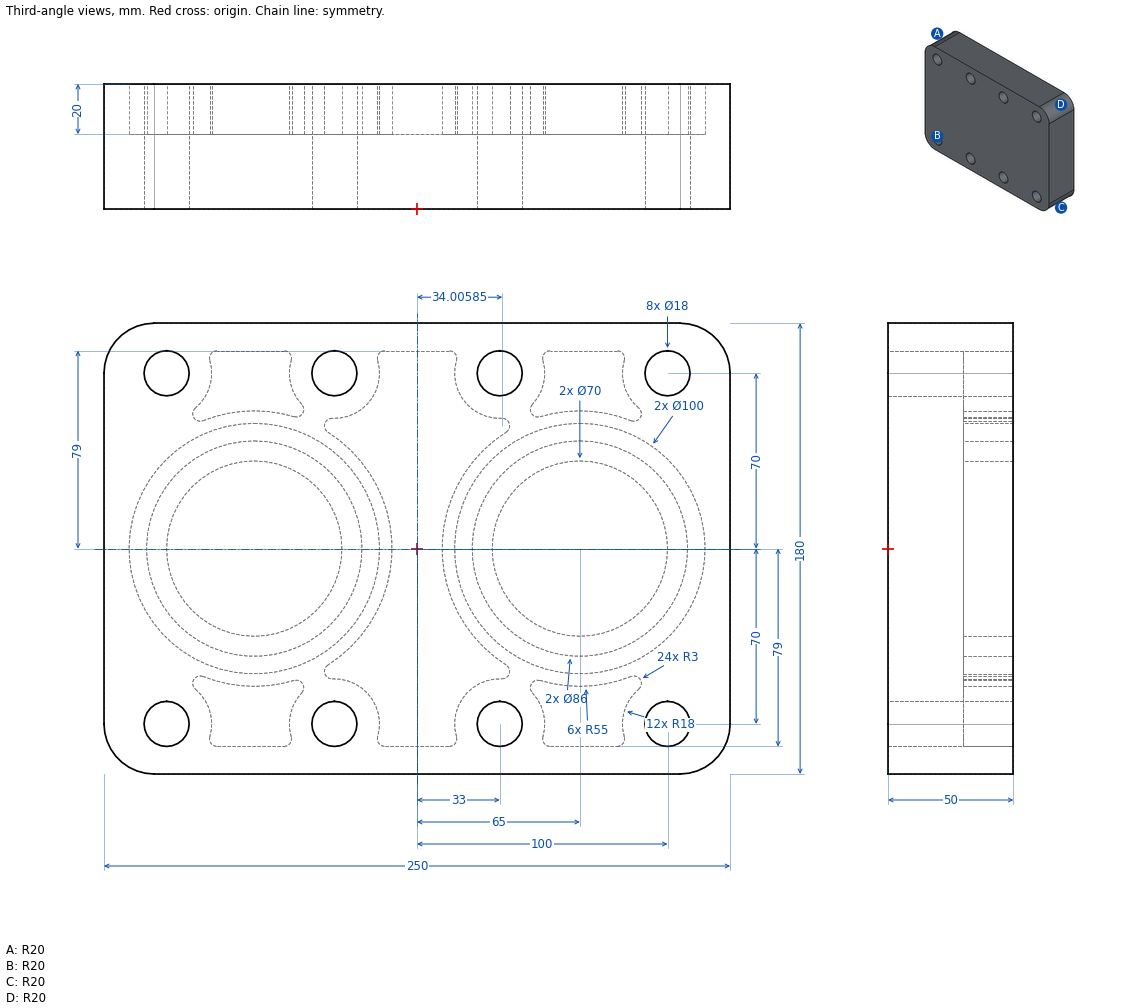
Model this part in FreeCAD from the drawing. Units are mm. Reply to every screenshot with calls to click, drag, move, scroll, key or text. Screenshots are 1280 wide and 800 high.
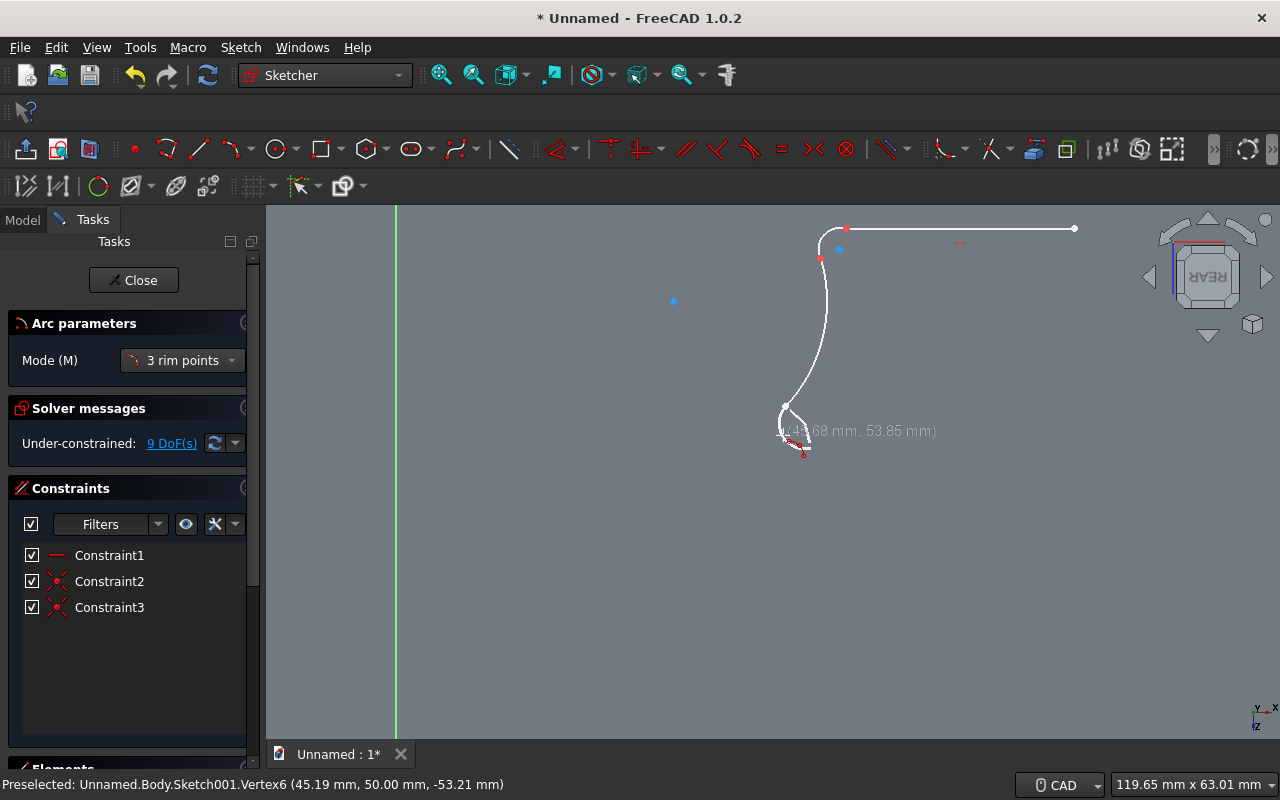
click(783, 435)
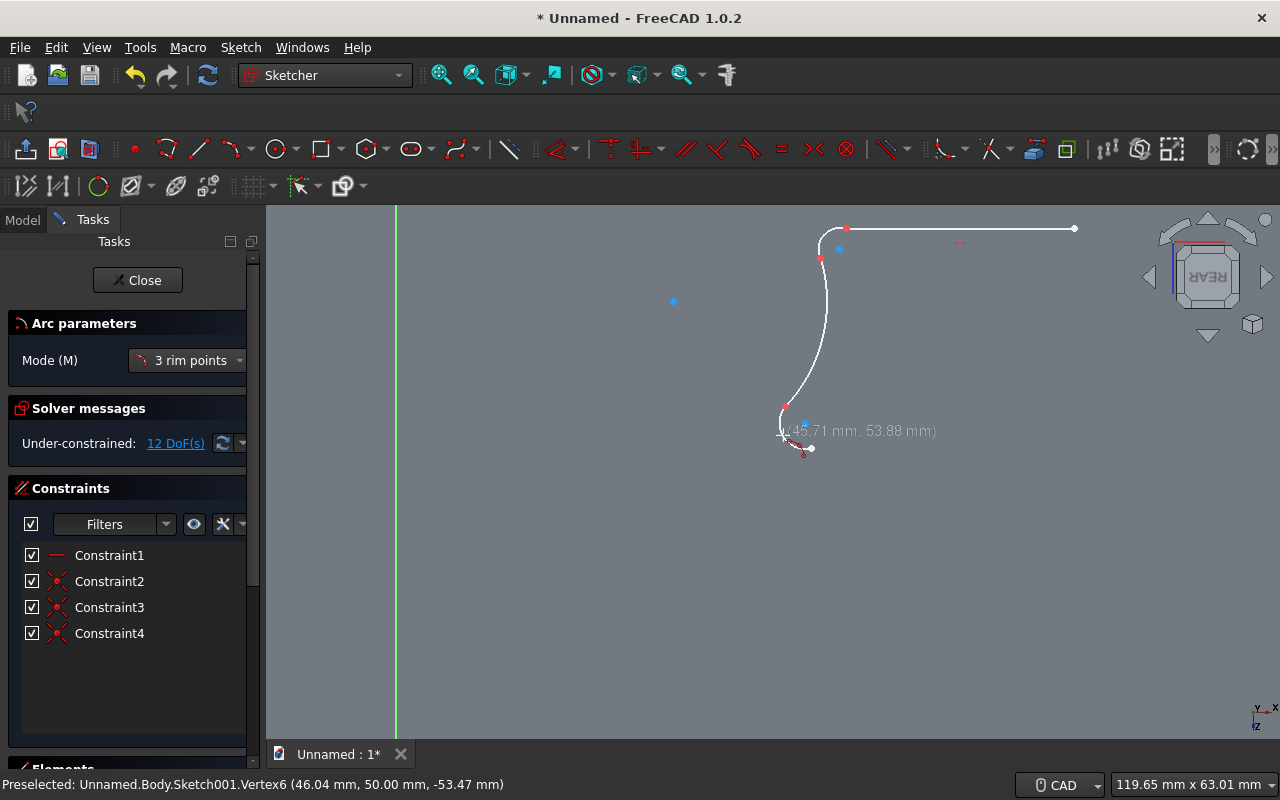
click(811, 448)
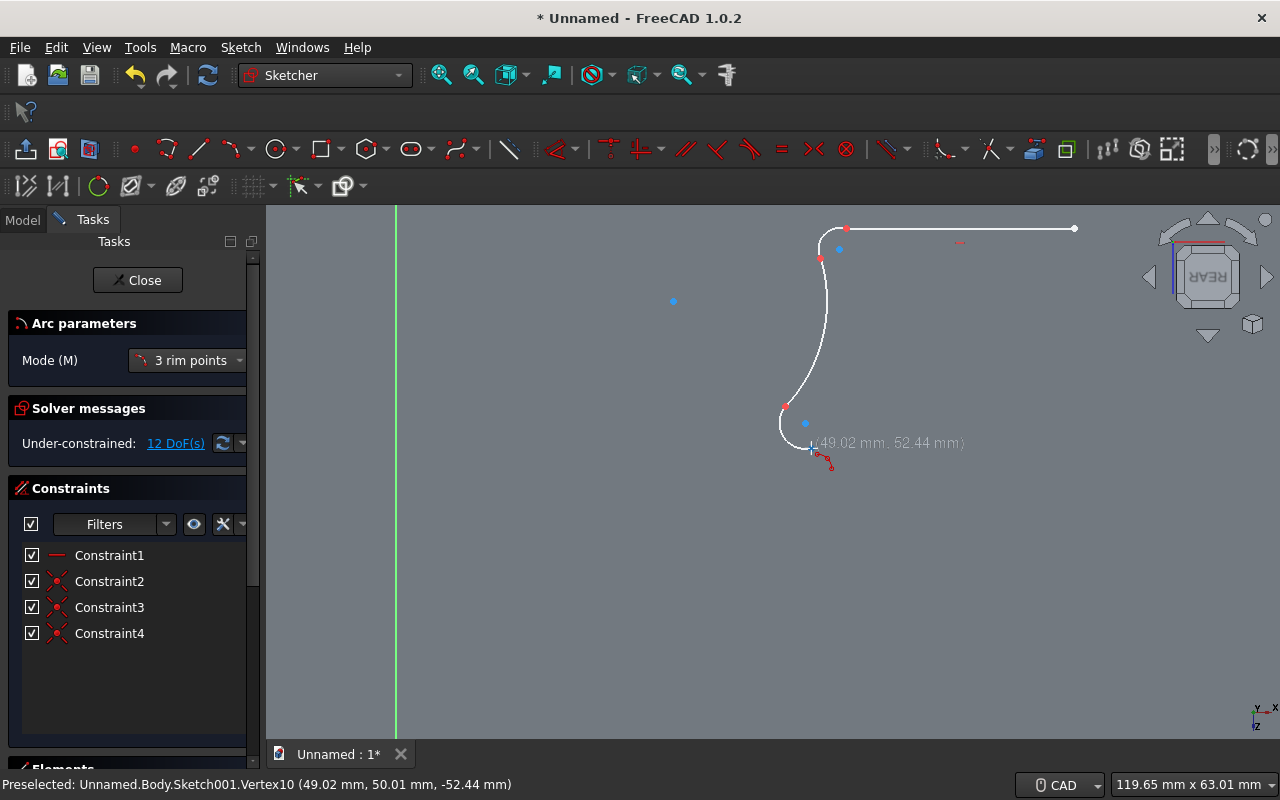
scroll(806, 334, down, 7)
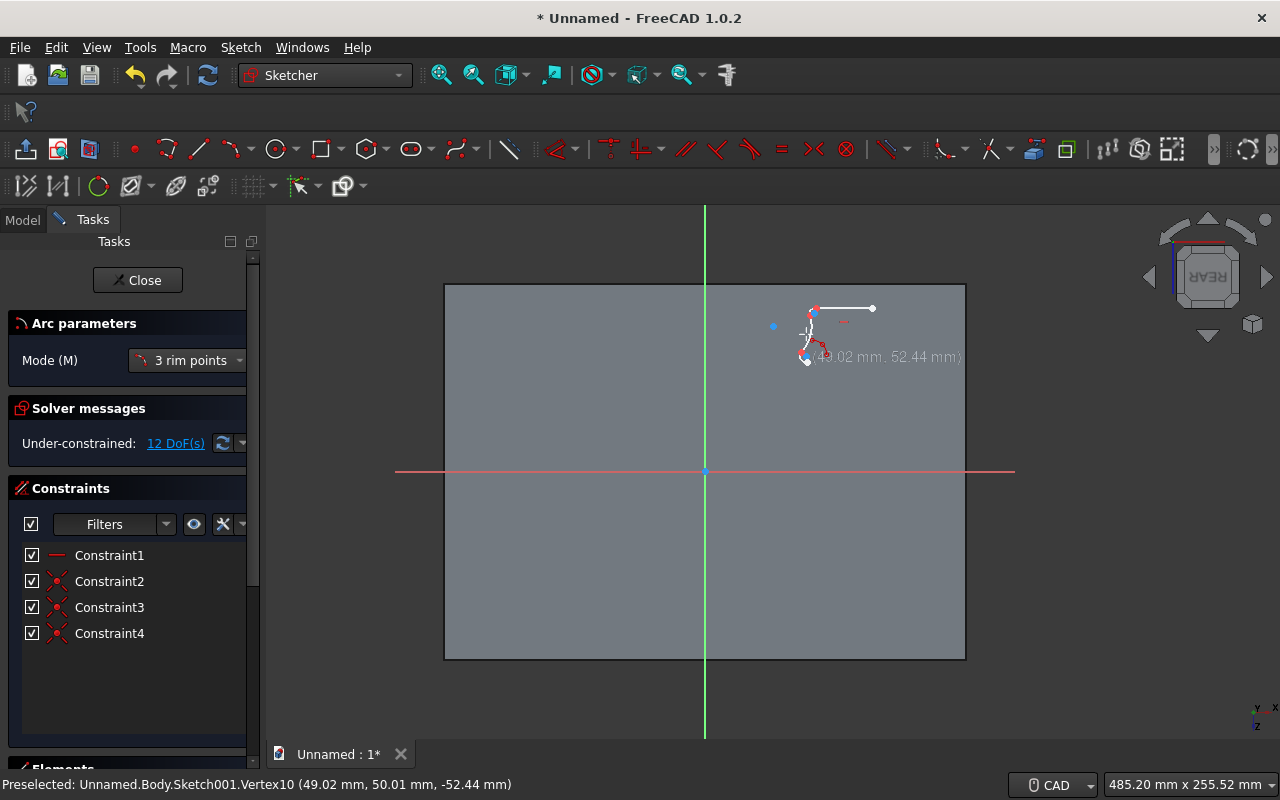
click(884, 365)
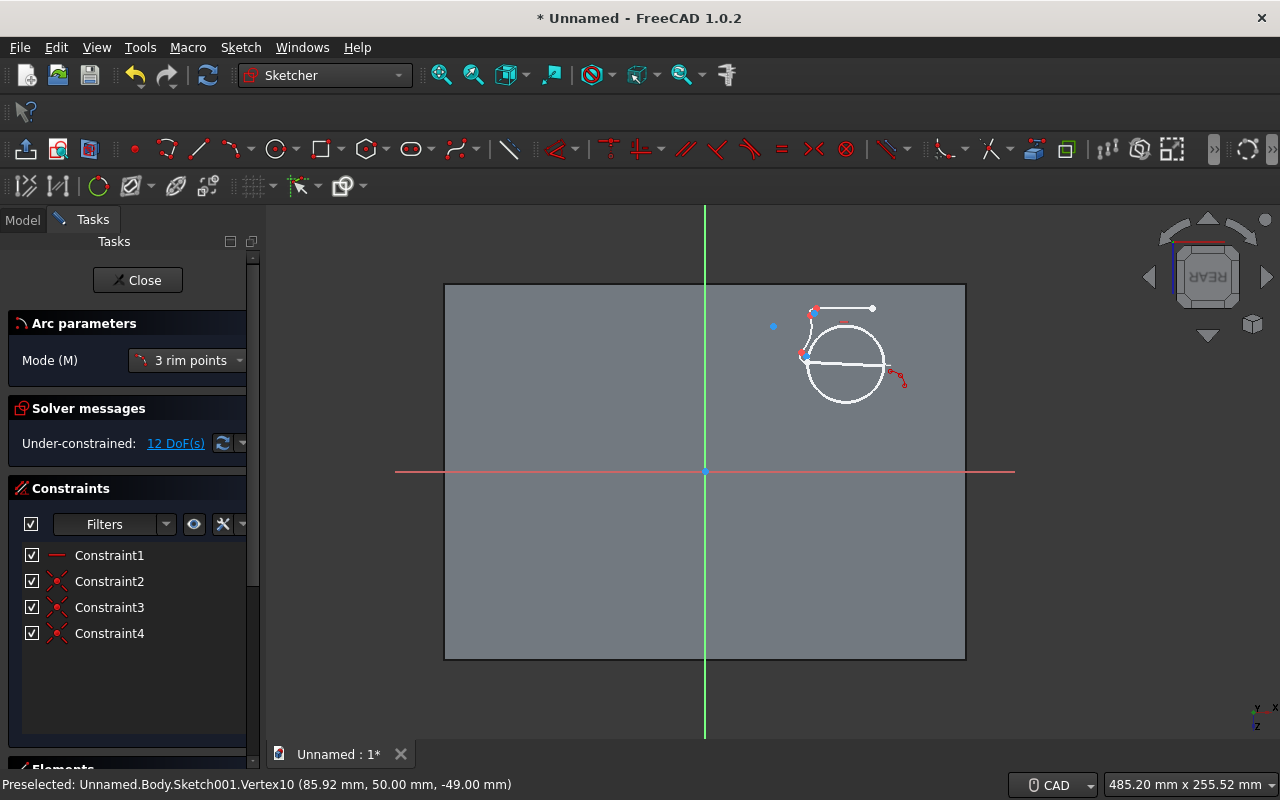
scroll(846, 357, up, 5)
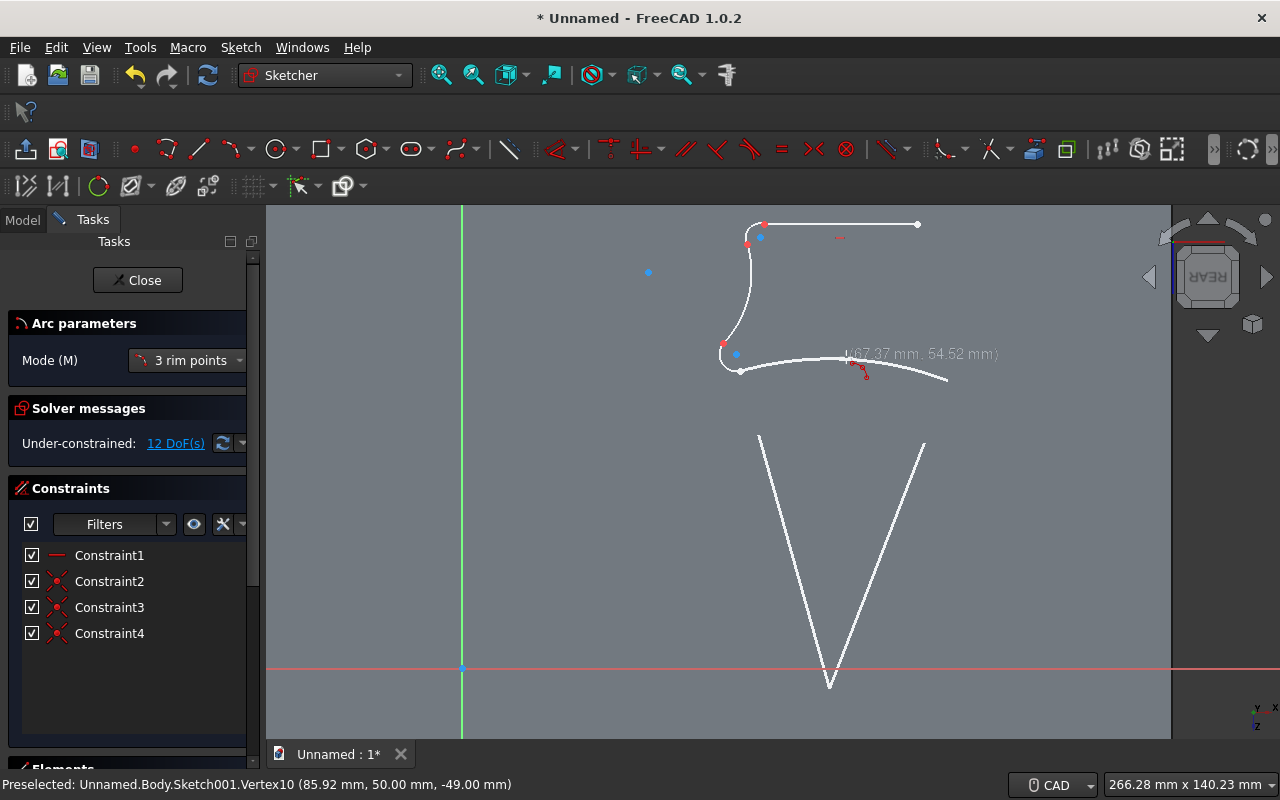
click(845, 357)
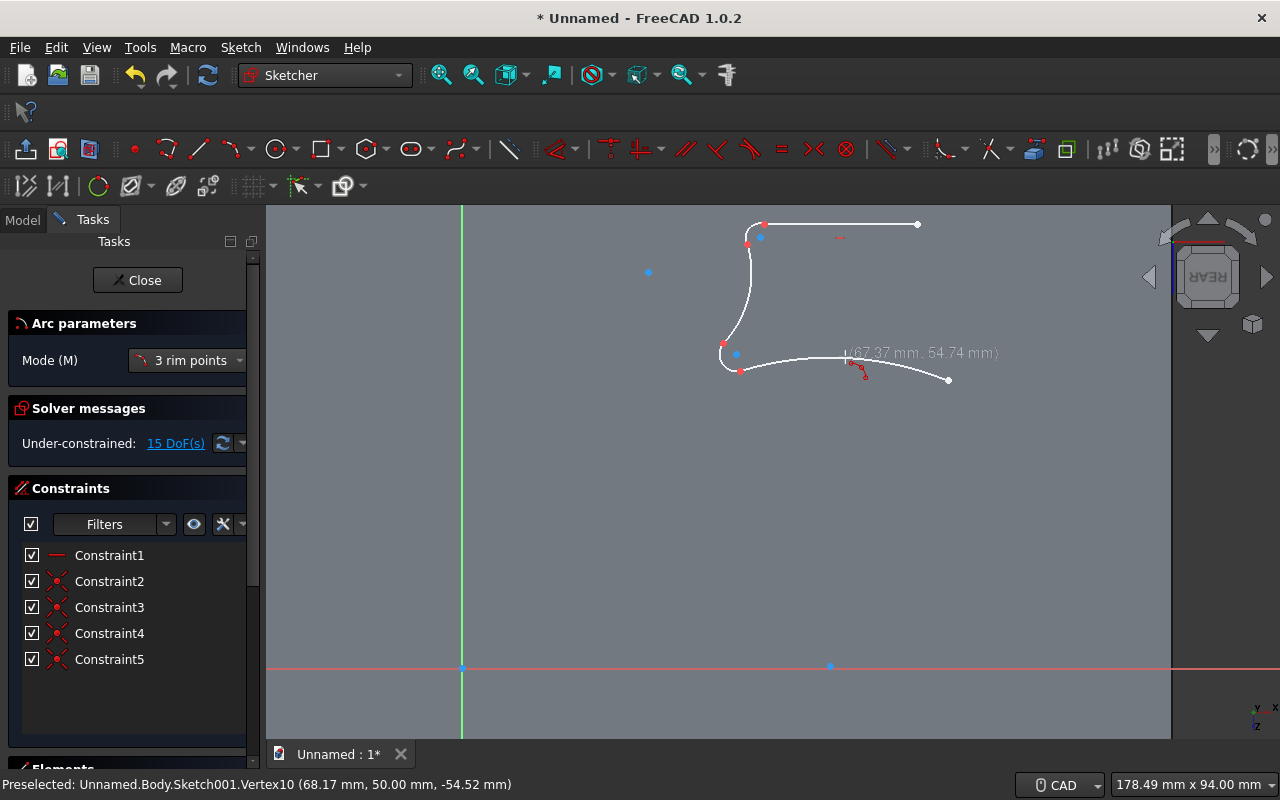
click(948, 381)
click(965, 350)
click(969, 372)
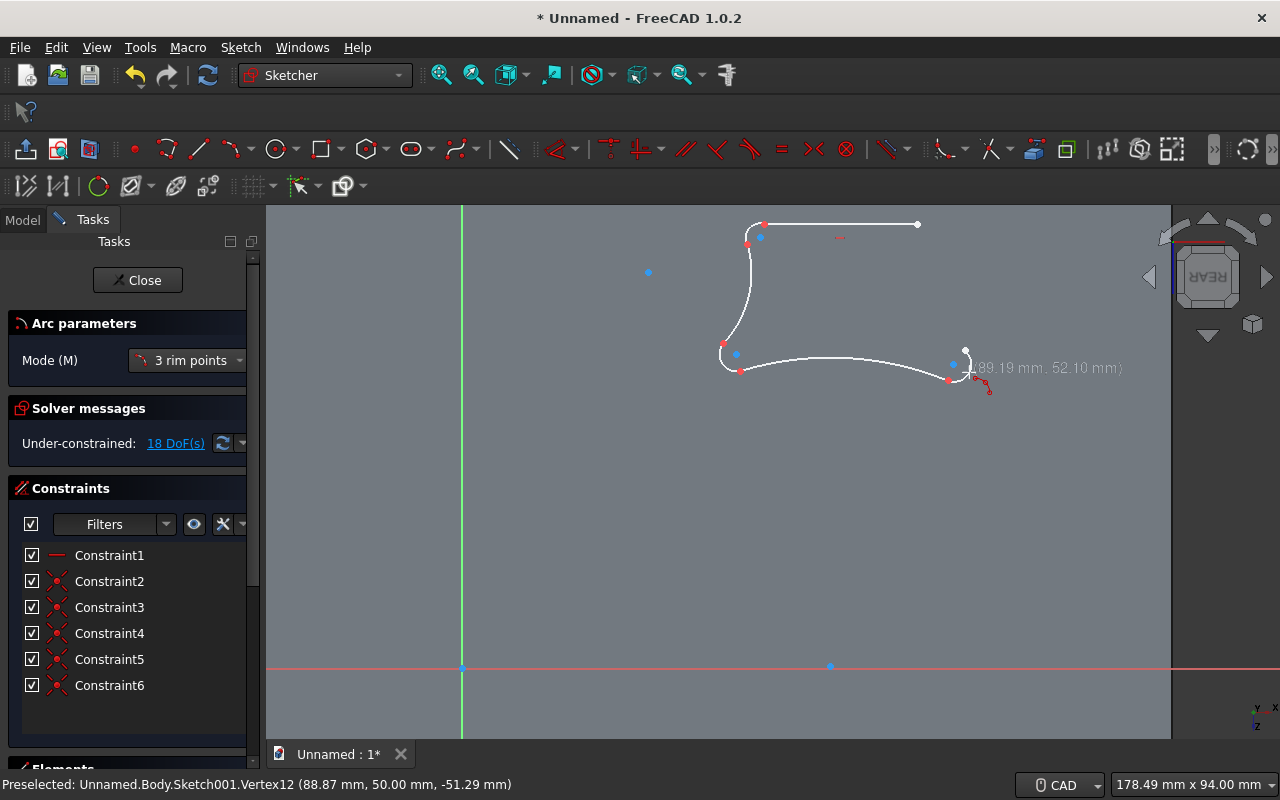
click(965, 351)
click(932, 242)
click(933, 301)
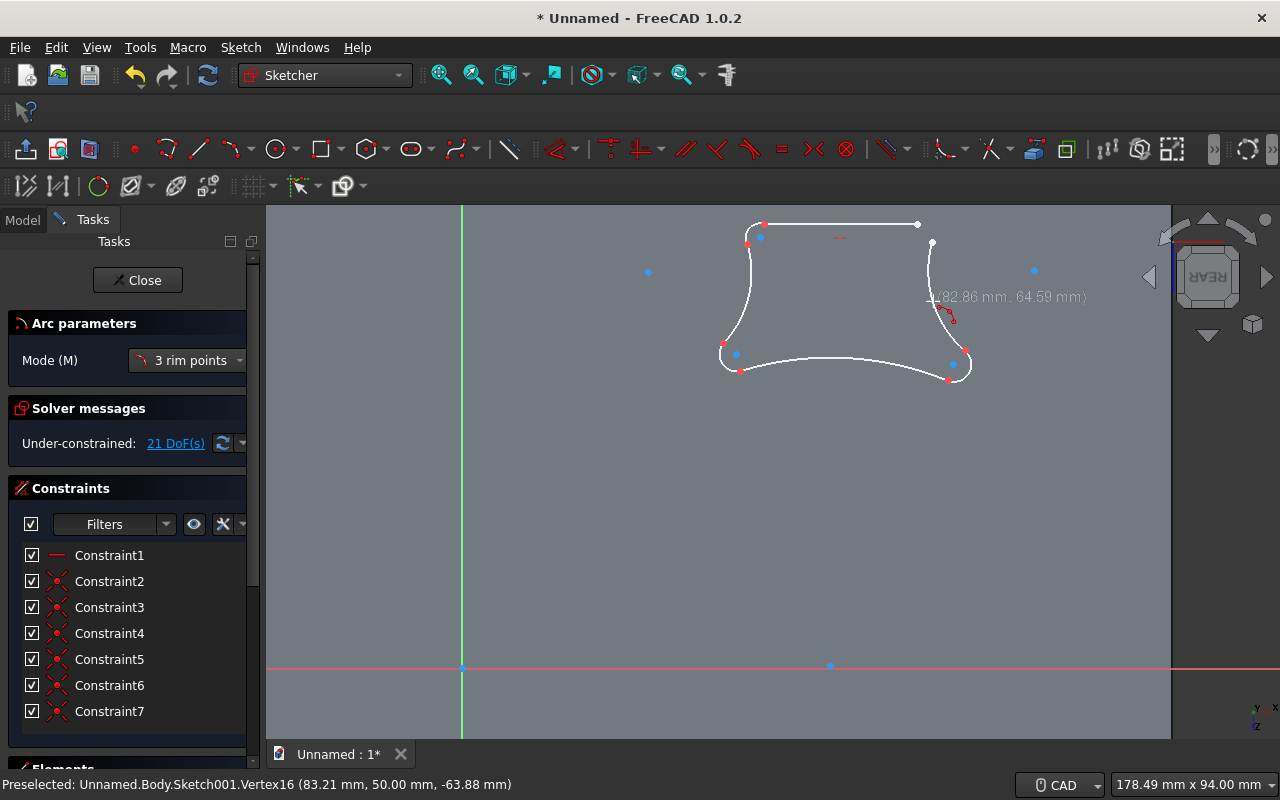
click(932, 243)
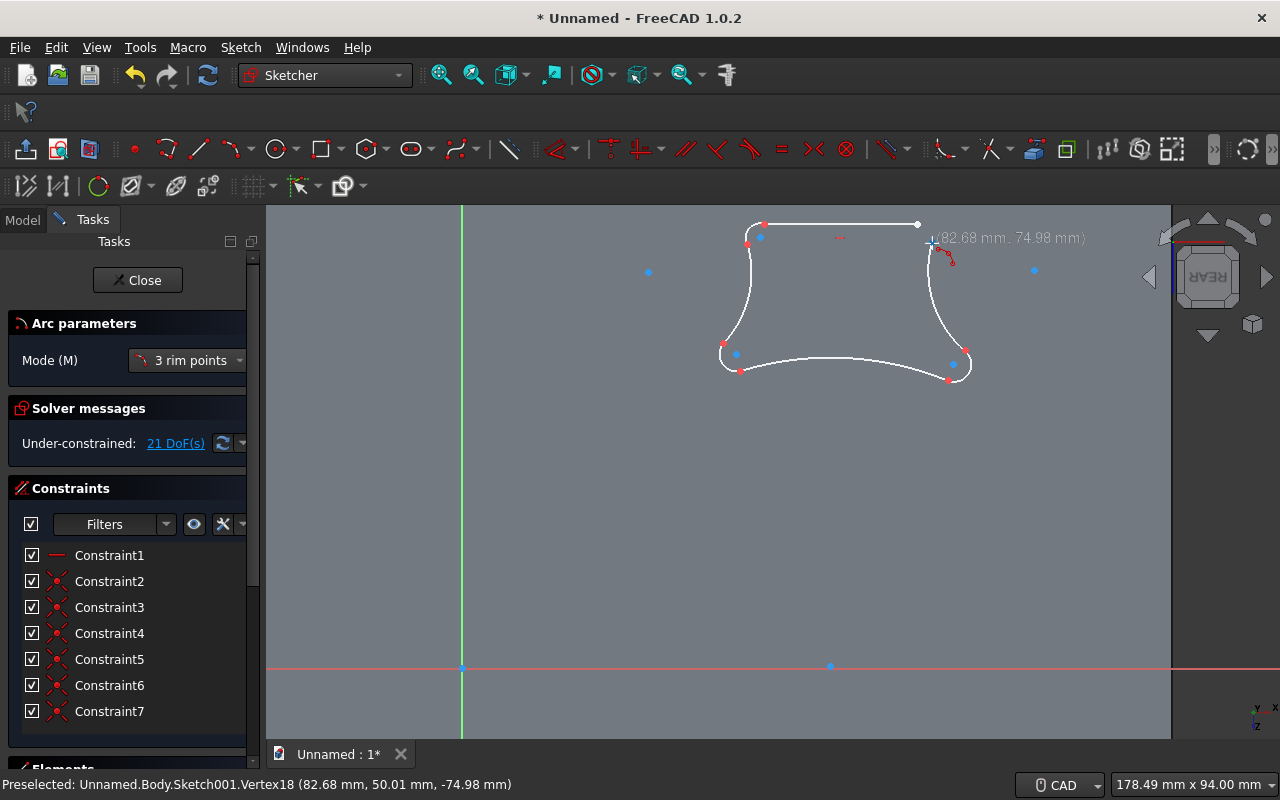
scroll(845, 357, down, 5)